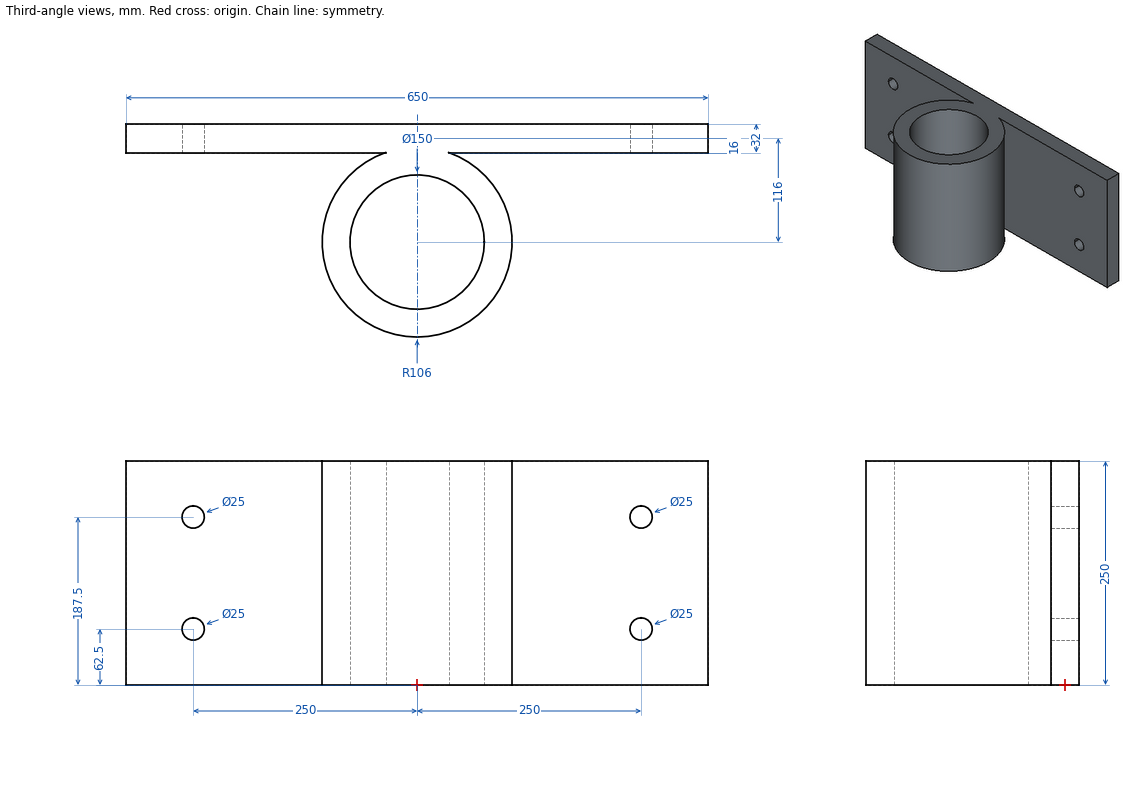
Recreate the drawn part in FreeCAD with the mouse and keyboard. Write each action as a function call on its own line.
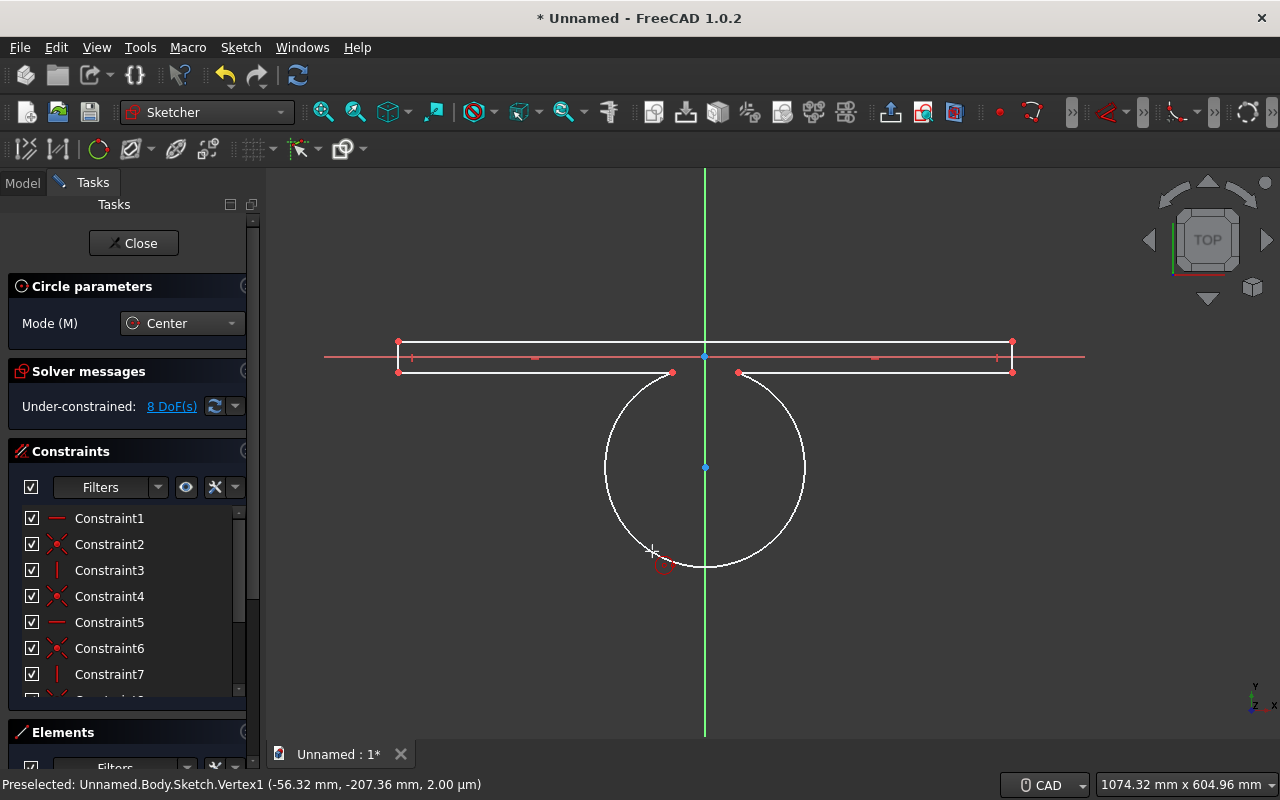
click(705, 466)
click(755, 416)
key(Escape)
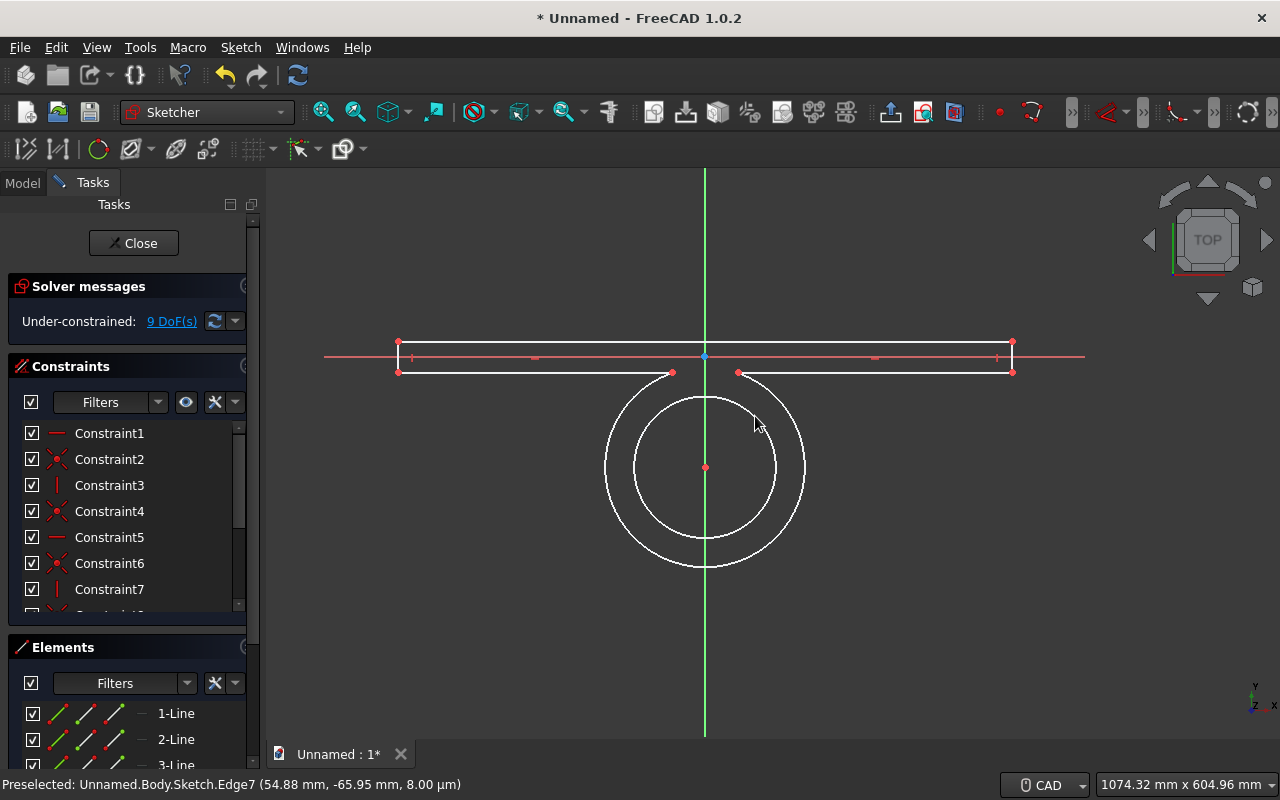
click(705, 467)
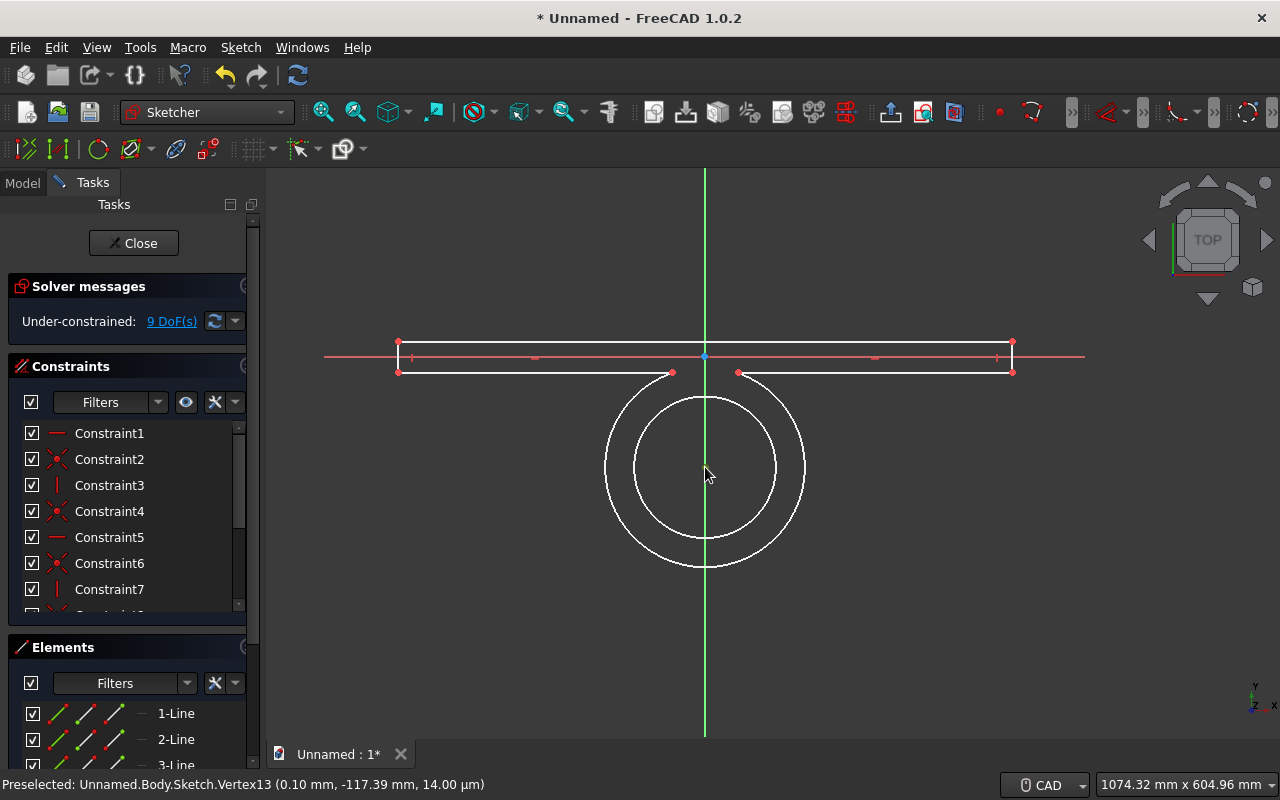
click(705, 674)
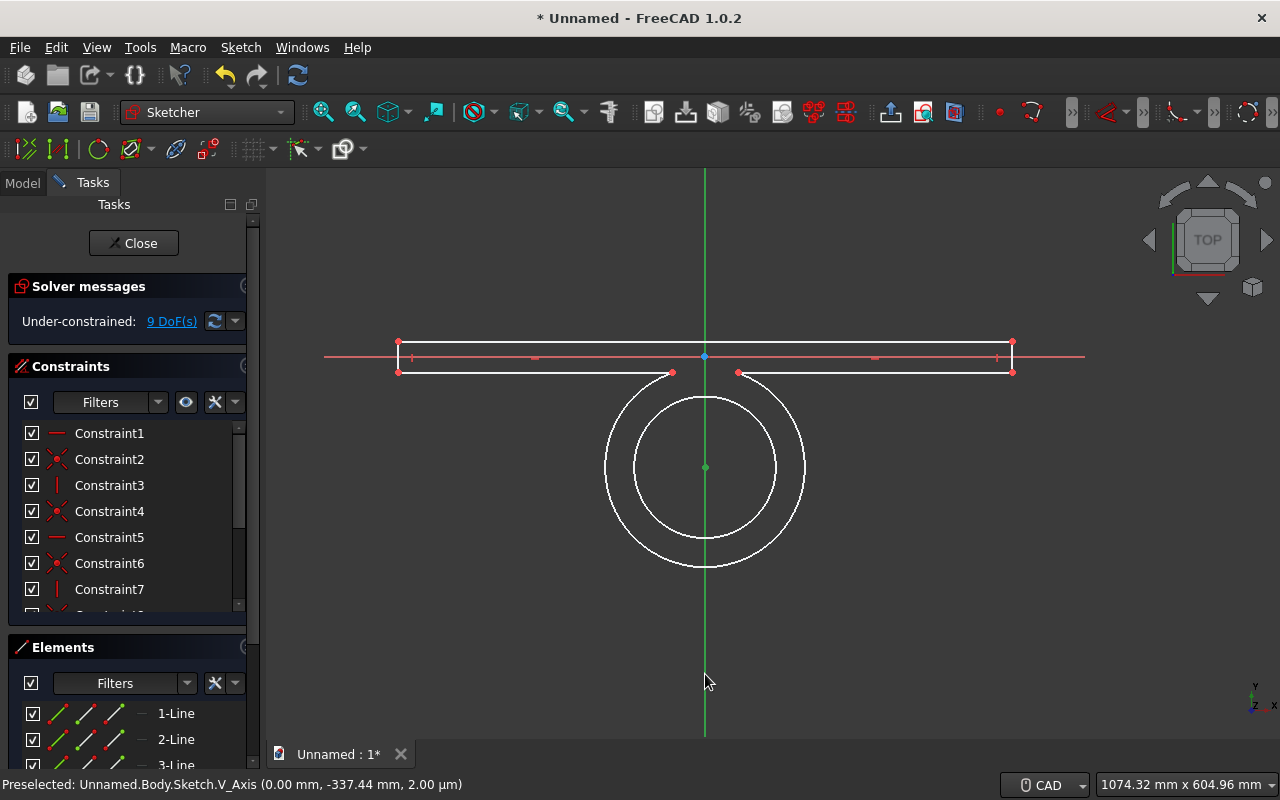
key(c)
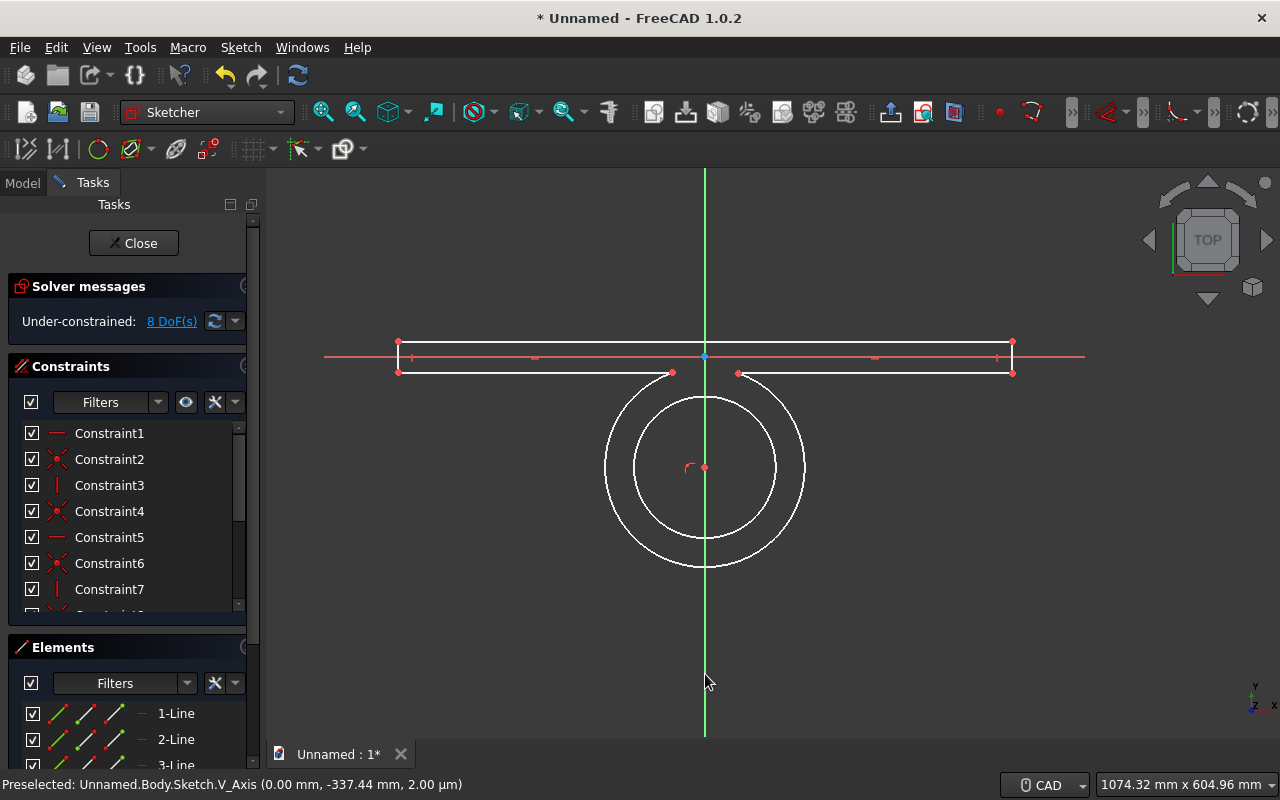
click(1012, 373)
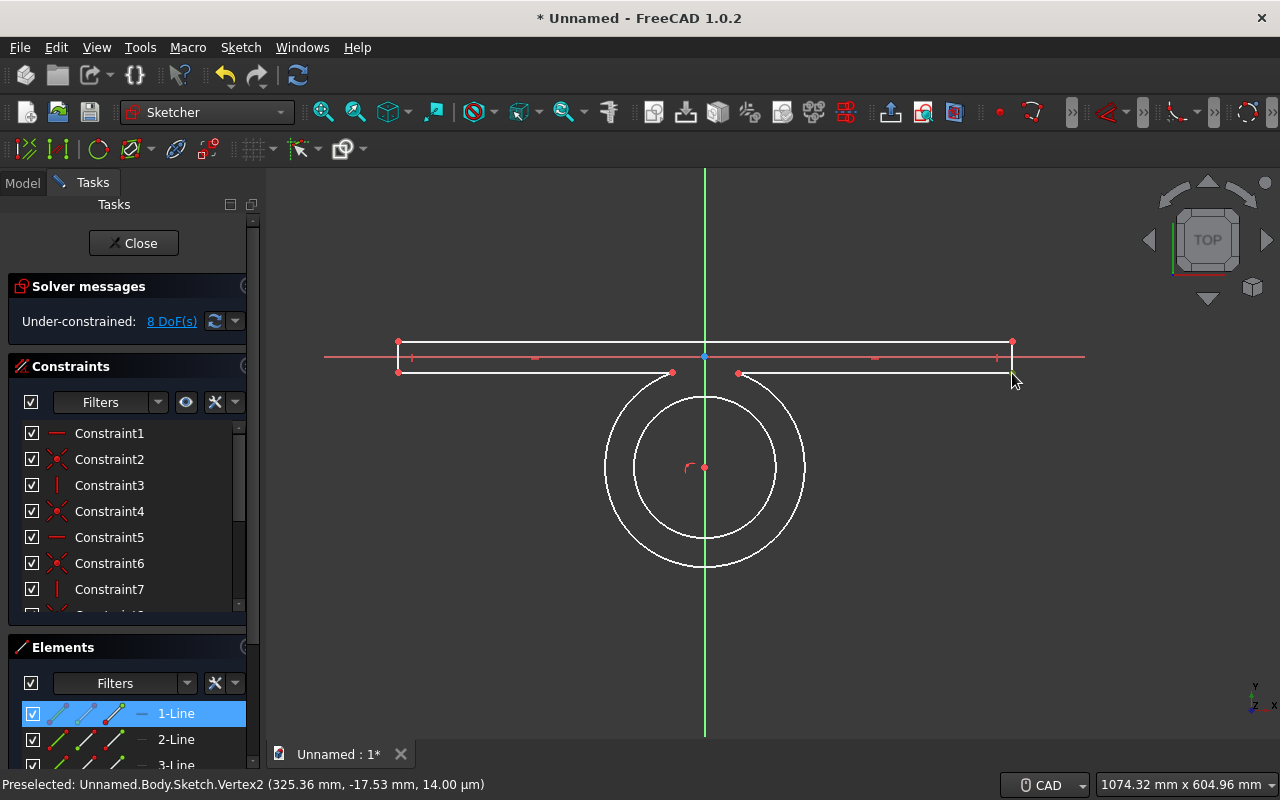
click(398, 373)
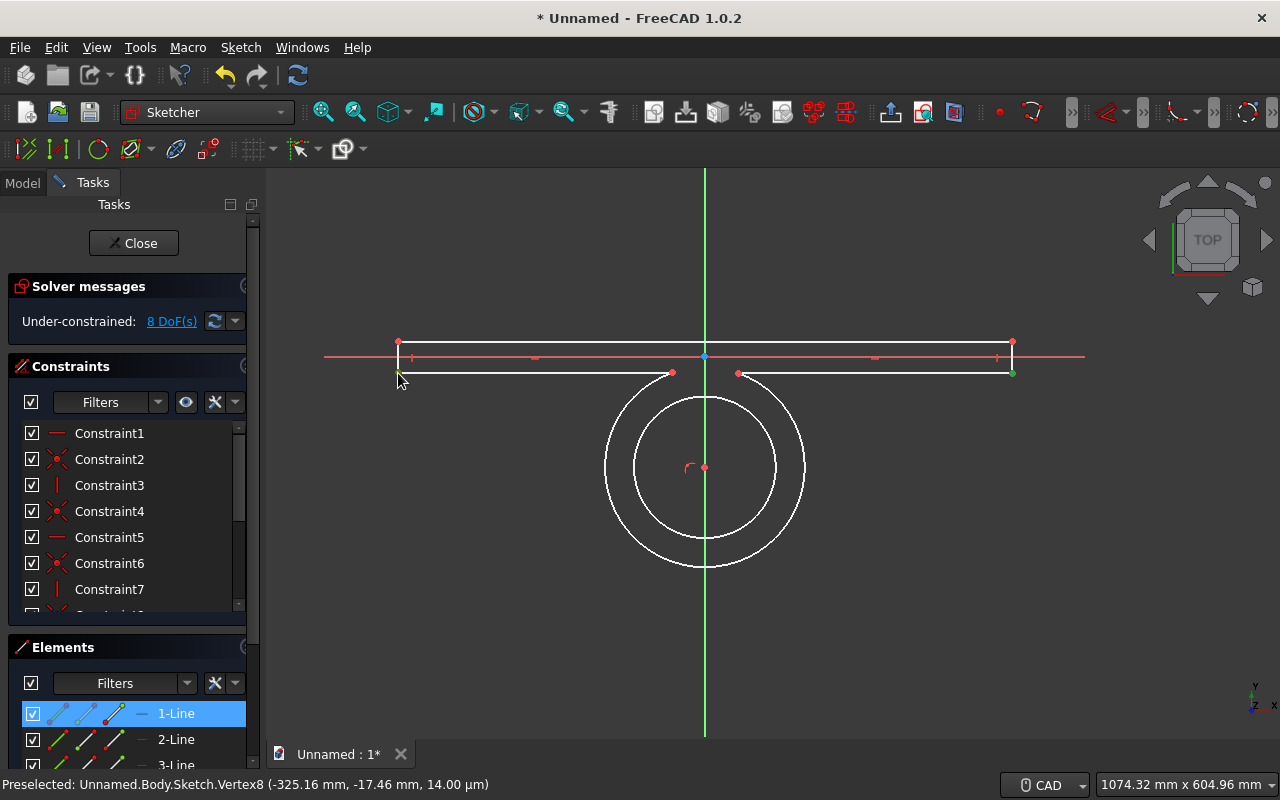
click(705, 674)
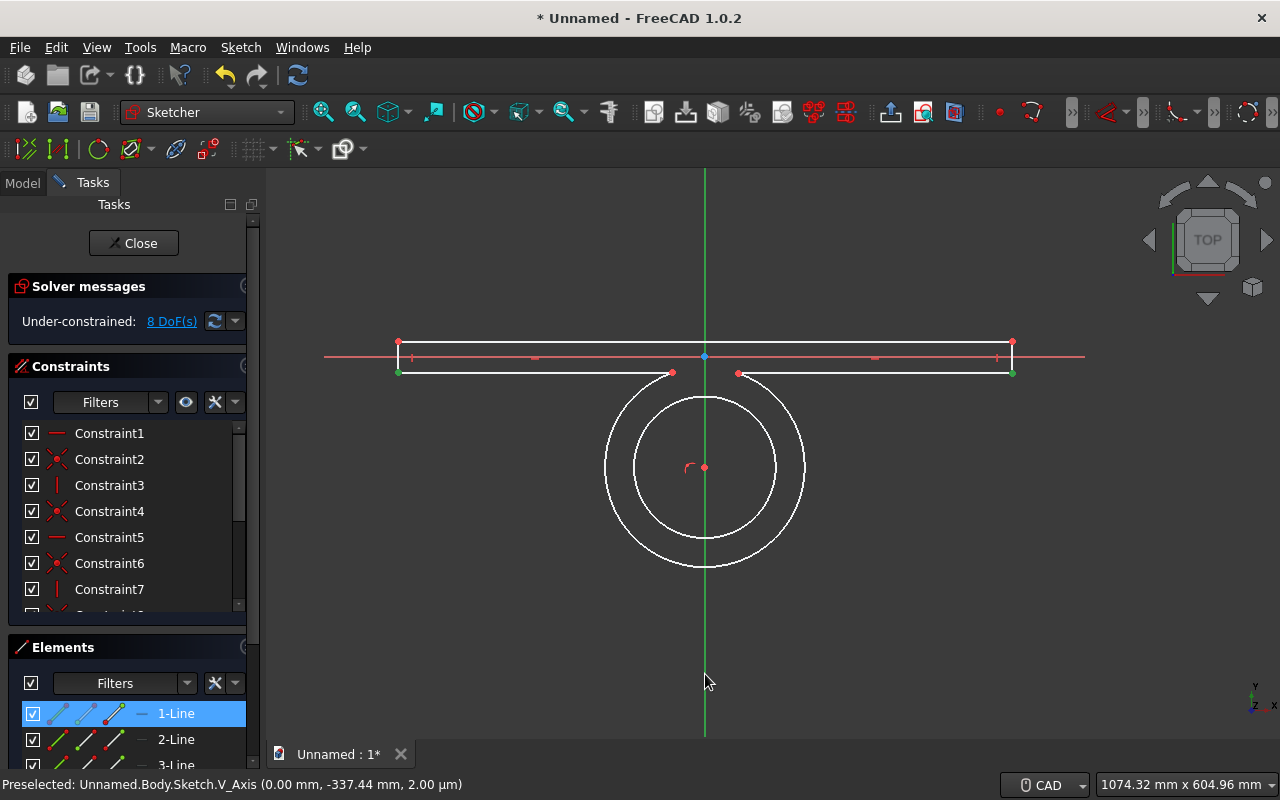
key(s)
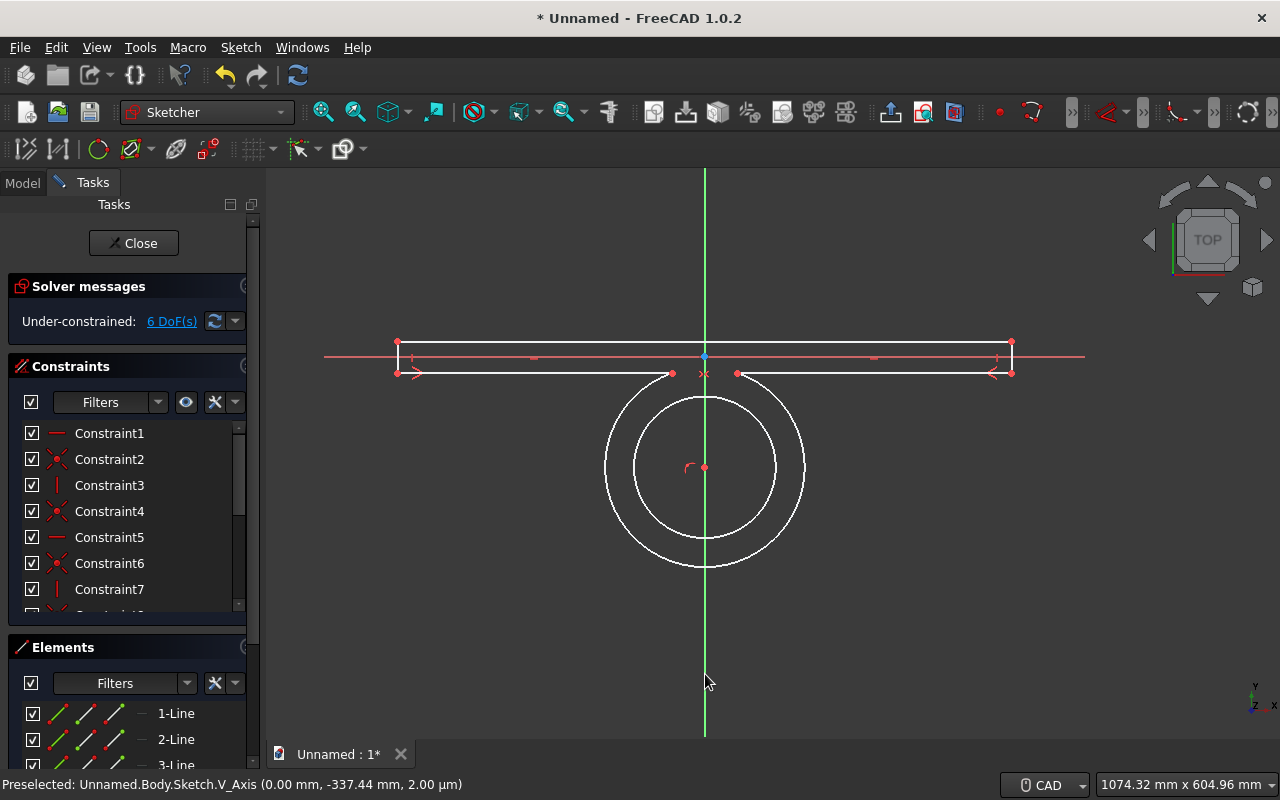
click(1106, 112)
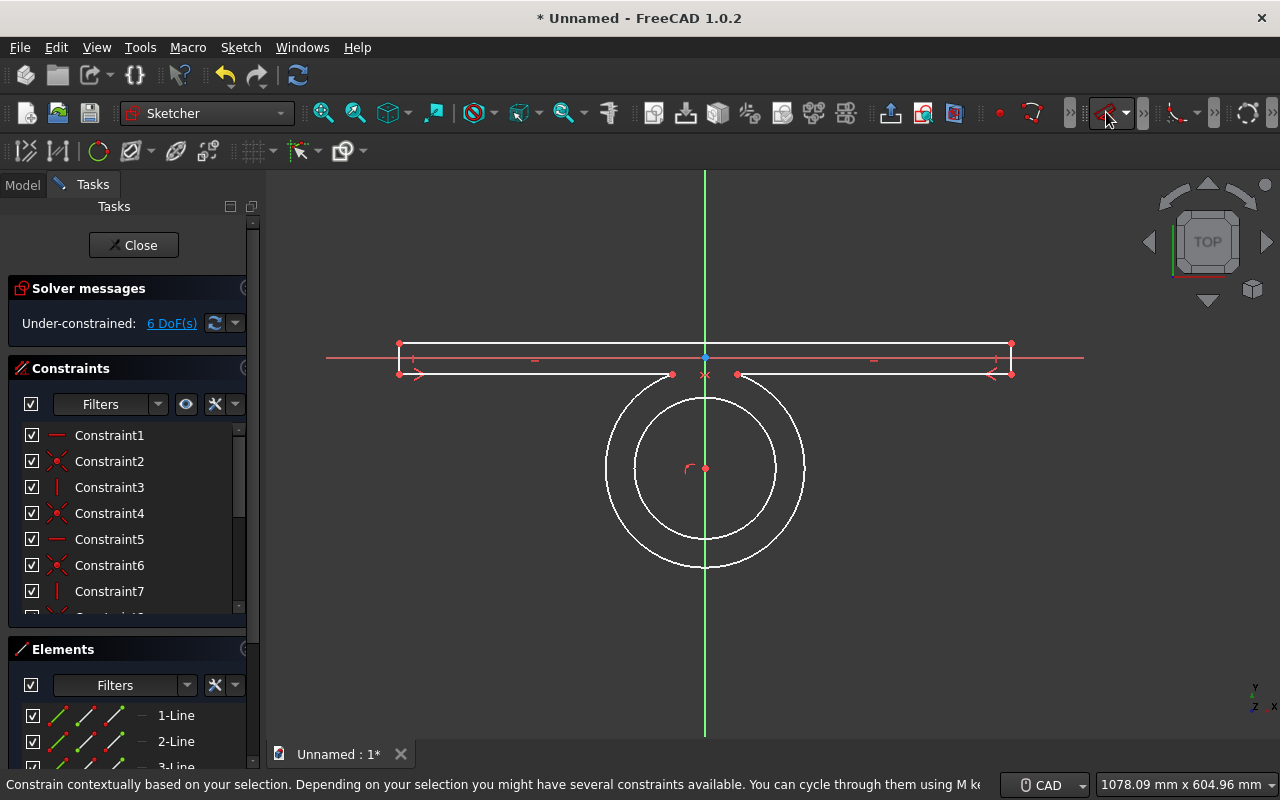
click(615, 511)
click(586, 525)